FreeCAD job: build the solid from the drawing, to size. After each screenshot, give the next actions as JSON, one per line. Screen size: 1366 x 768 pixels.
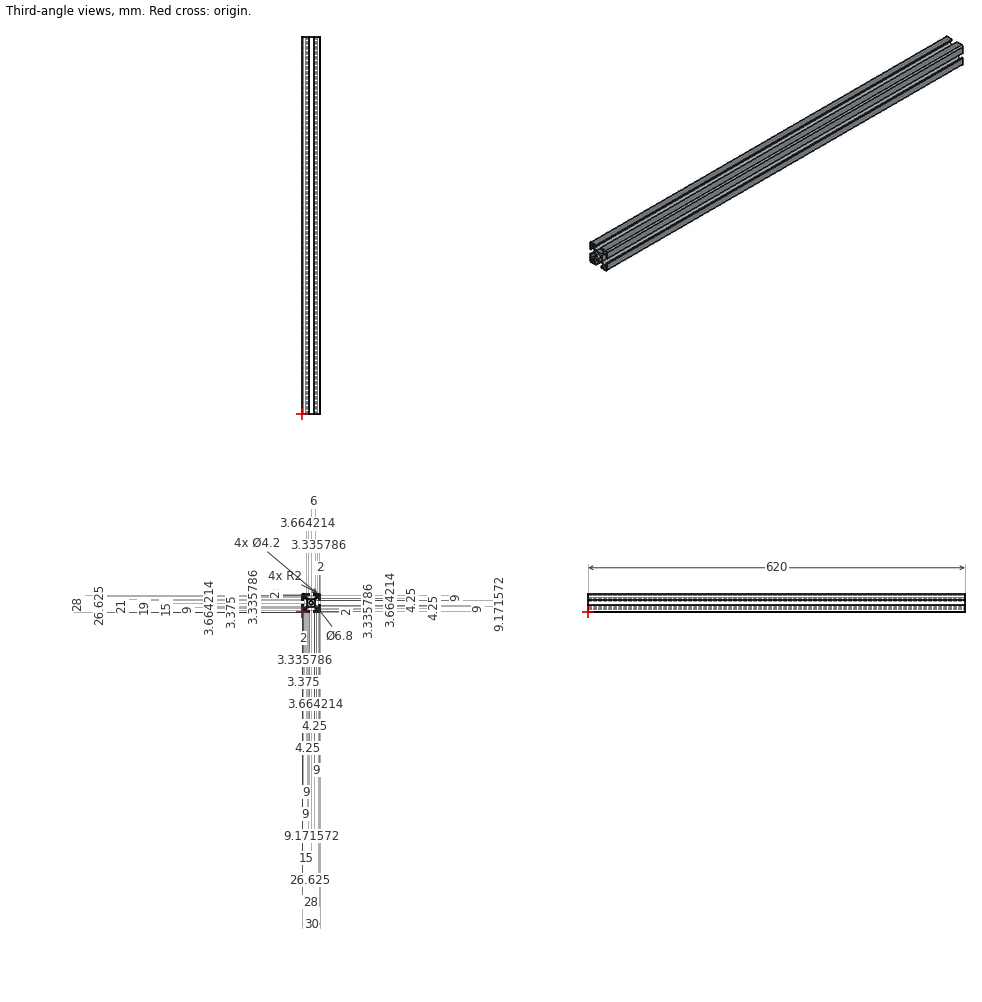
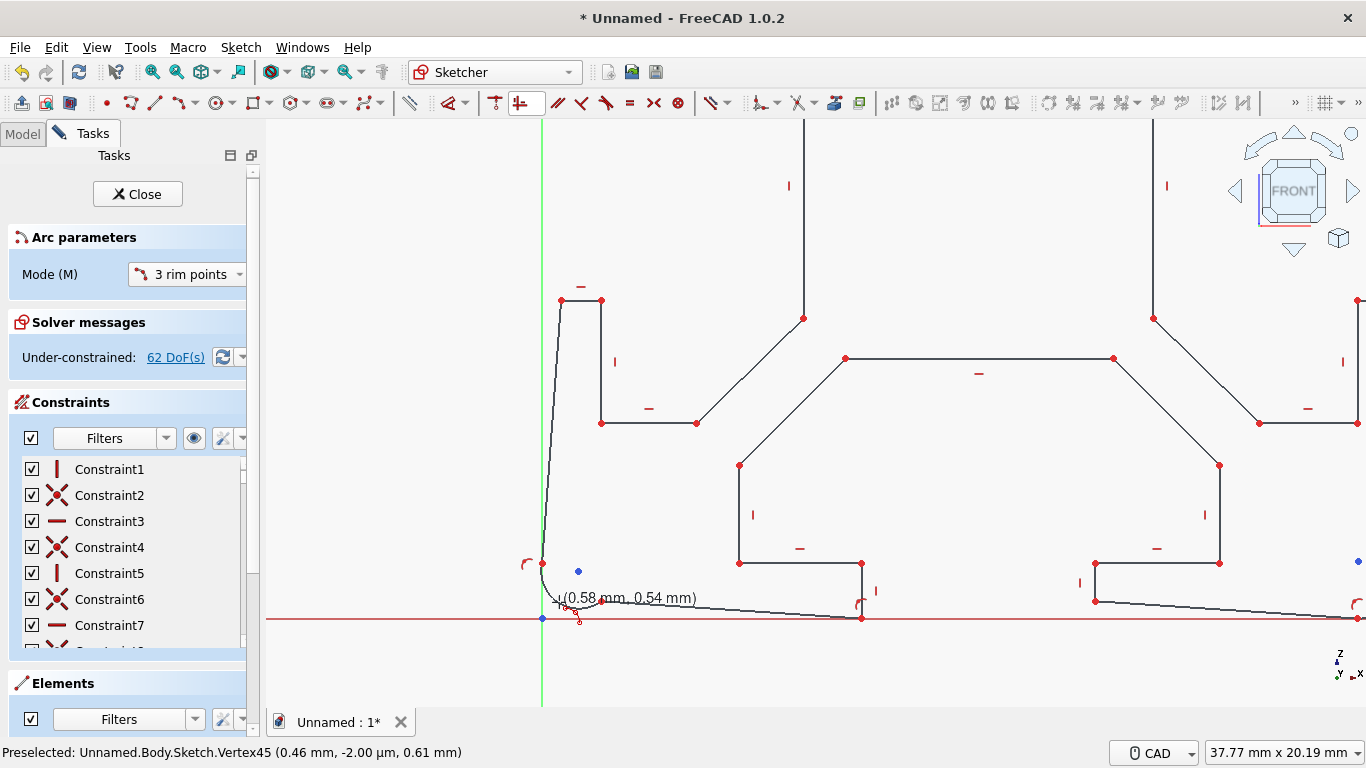
{"action": "scroll", "coordinate": [559, 602], "scroll_direction": "down", "scroll_amount": 4}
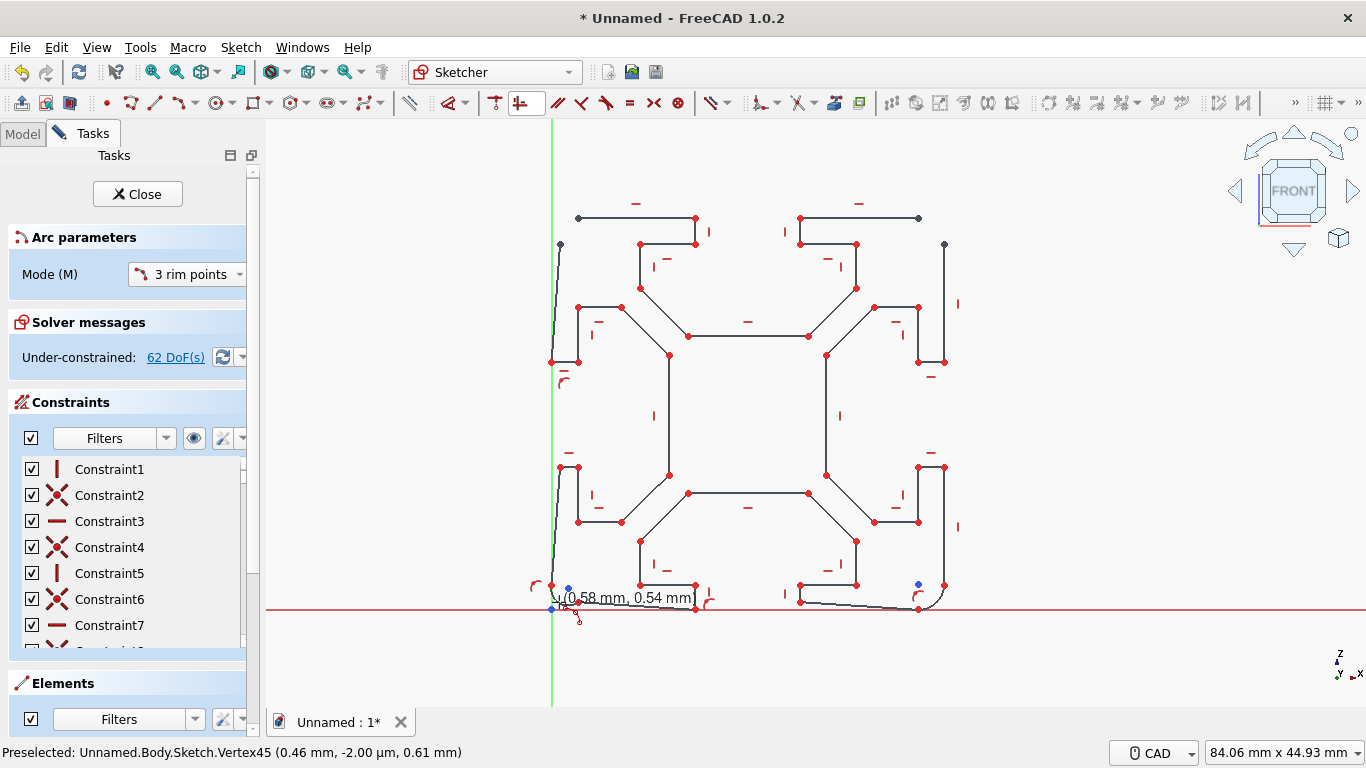
{"action": "left_click", "coordinate": [560, 244]}
{"action": "left_click", "coordinate": [578, 218]}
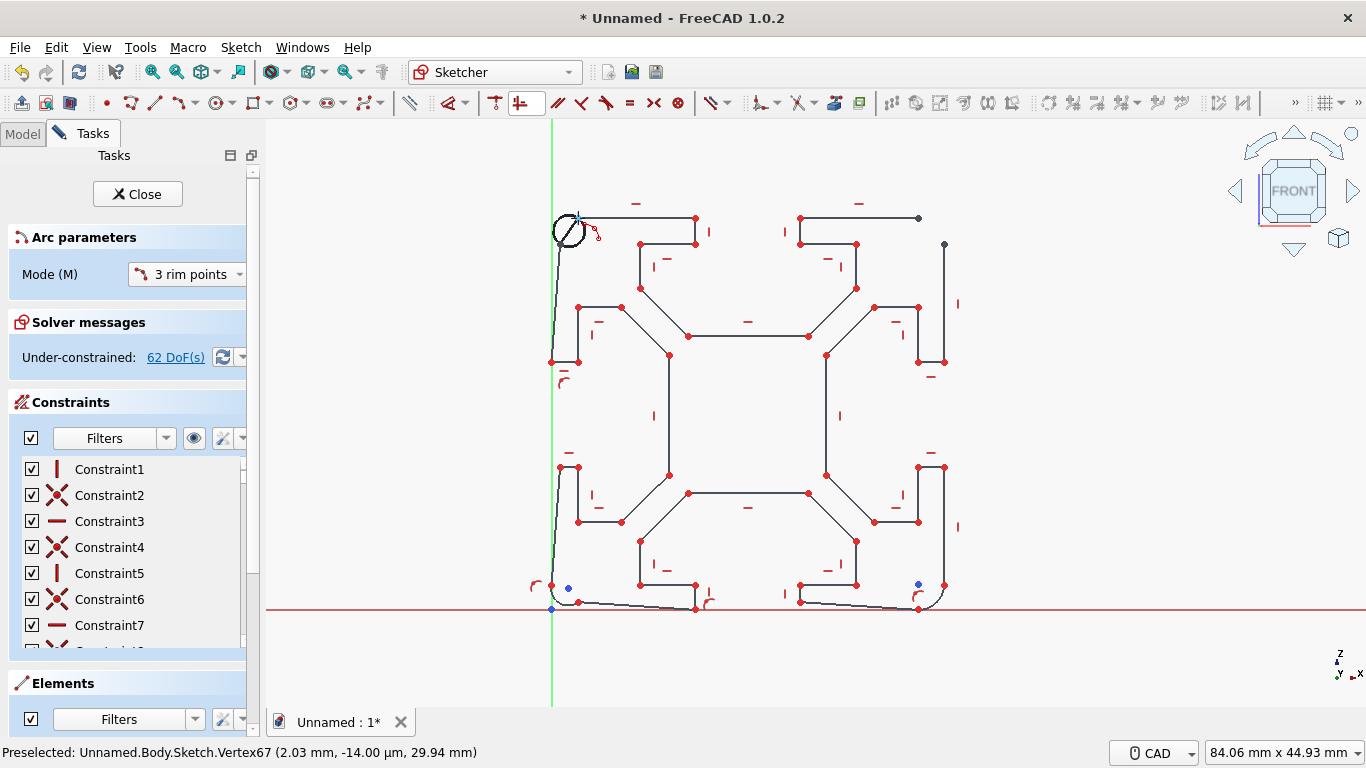
{"action": "scroll", "coordinate": [559, 225], "scroll_direction": "up", "scroll_amount": 4}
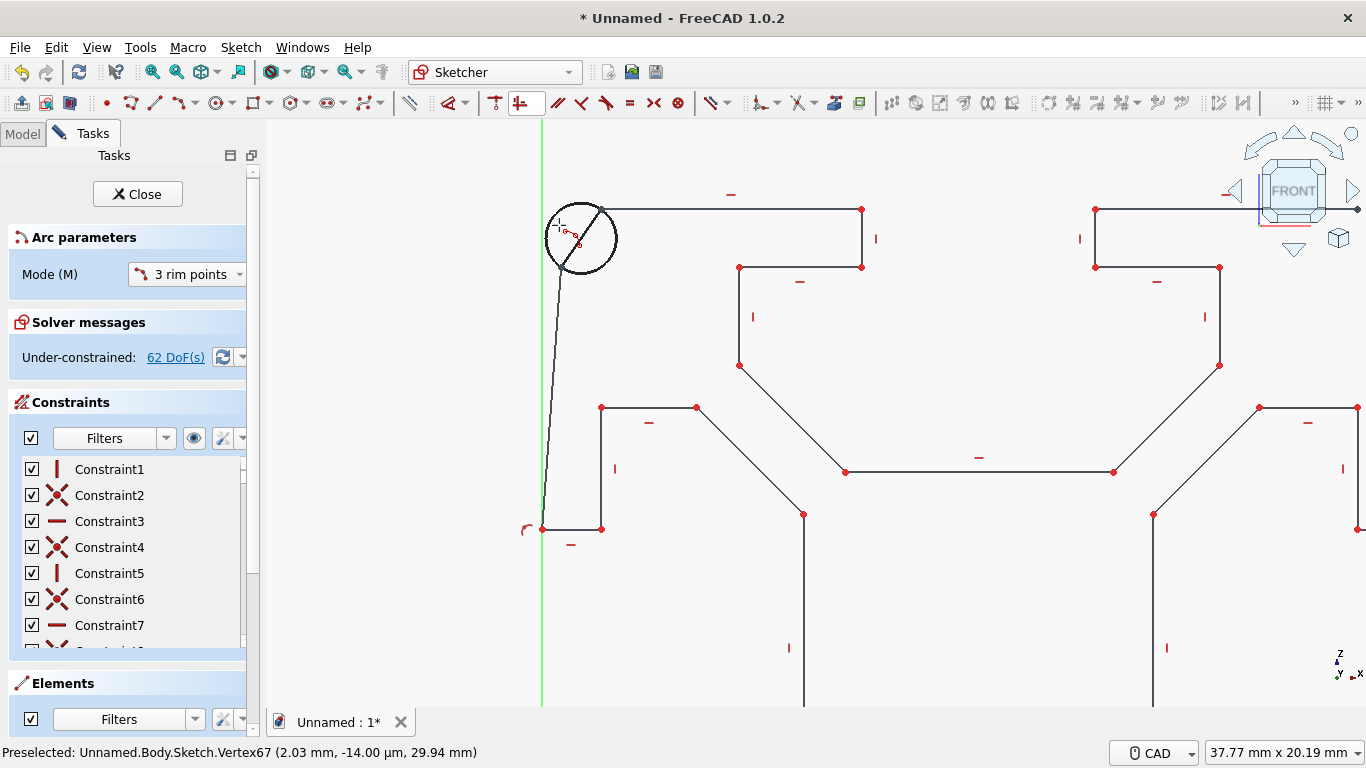
{"action": "left_click", "coordinate": [559, 225]}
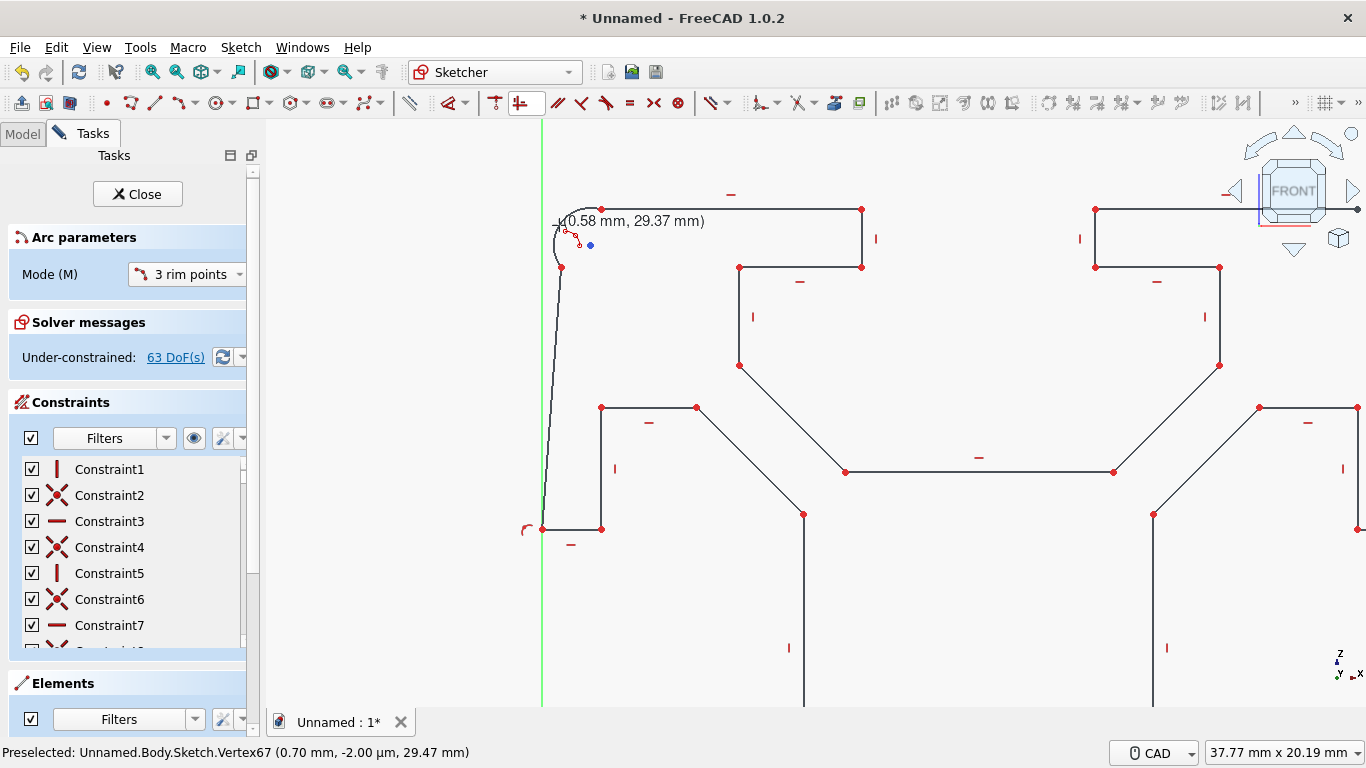
{"action": "scroll", "coordinate": [559, 224], "scroll_direction": "down", "scroll_amount": 4}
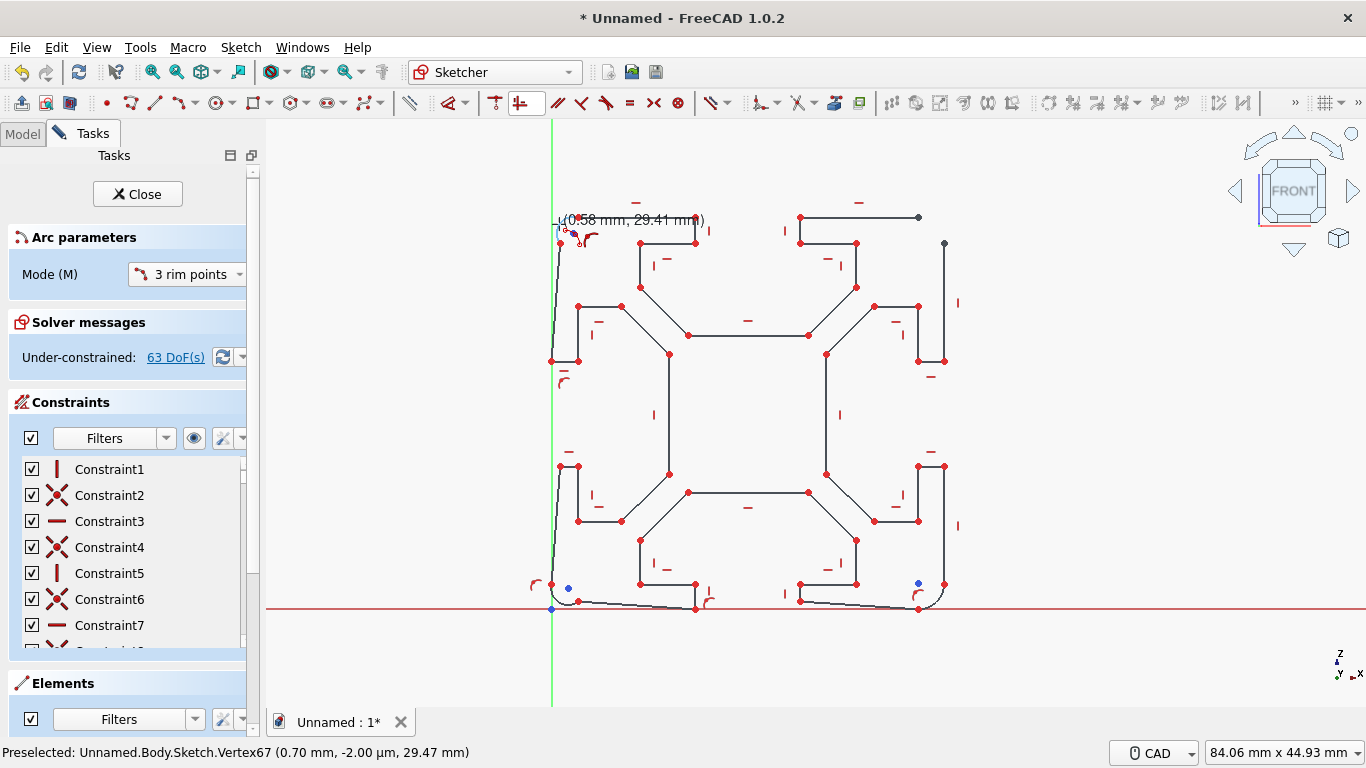
{"action": "left_click", "coordinate": [918, 218]}
{"action": "left_click", "coordinate": [944, 244]}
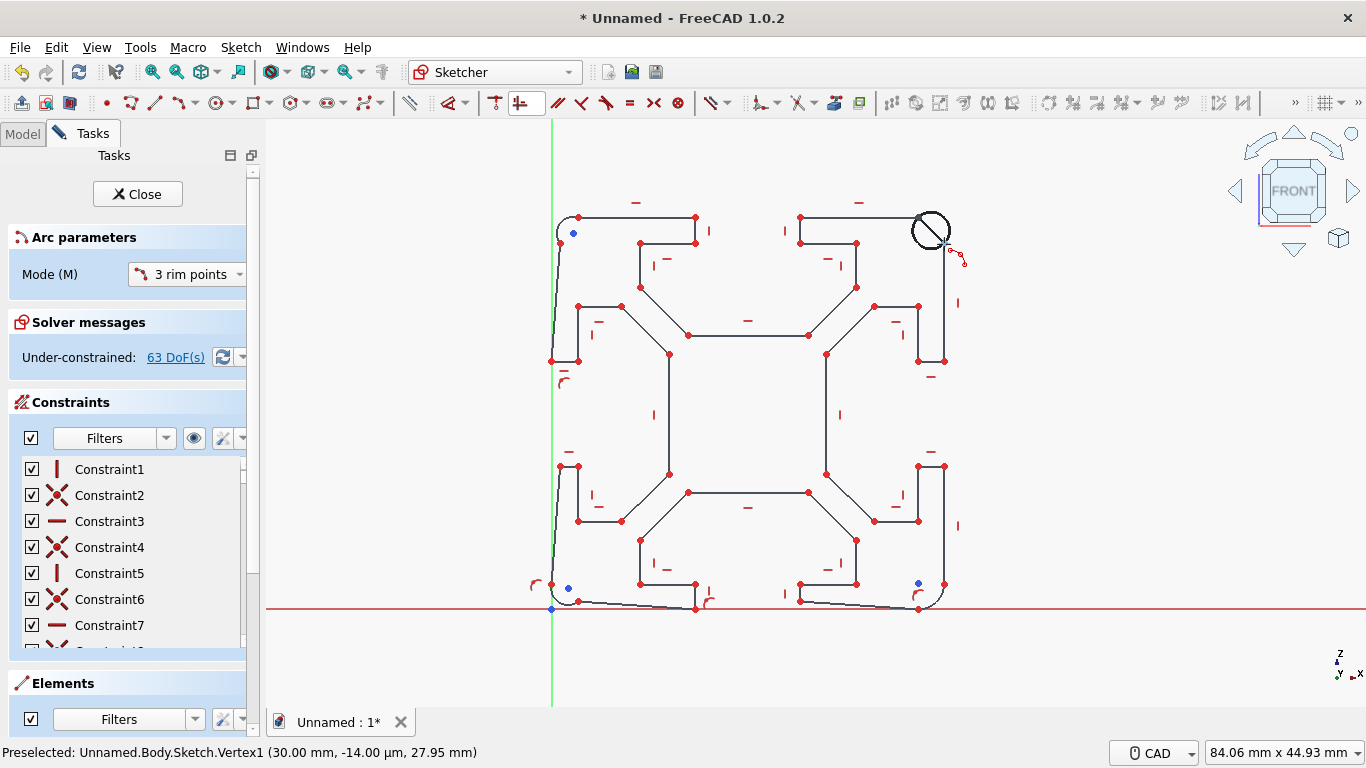
{"action": "scroll", "coordinate": [936, 224], "scroll_direction": "up", "scroll_amount": 4}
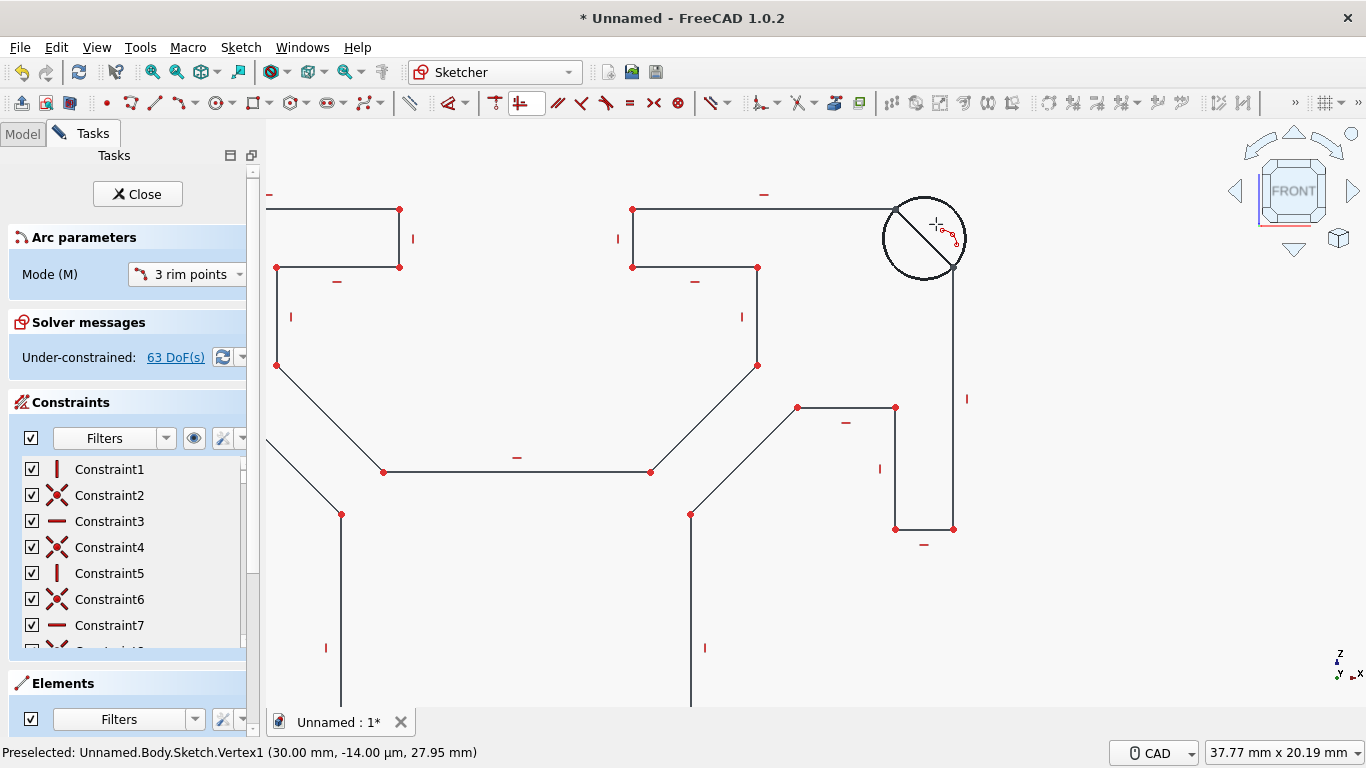
{"action": "left_click", "coordinate": [936, 225]}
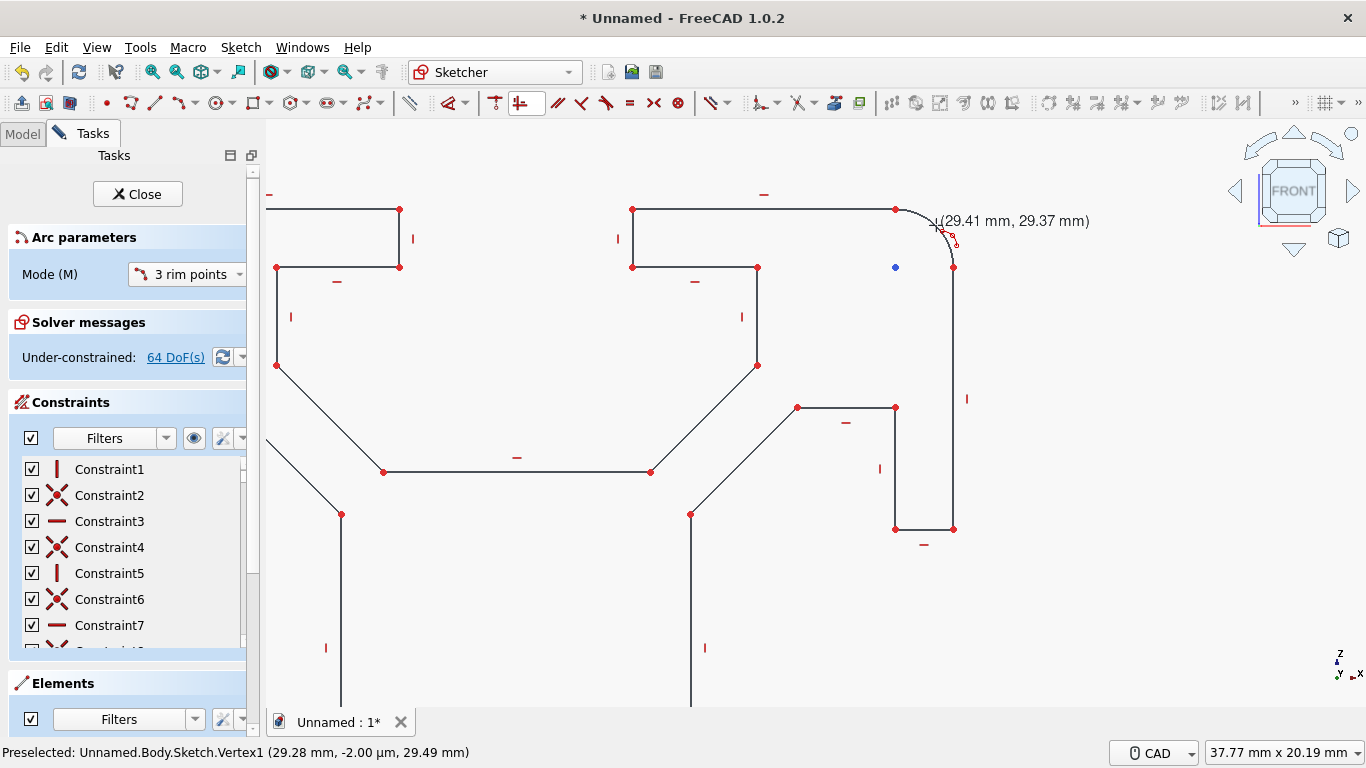
{"action": "left_click", "coordinate": [216, 104]}